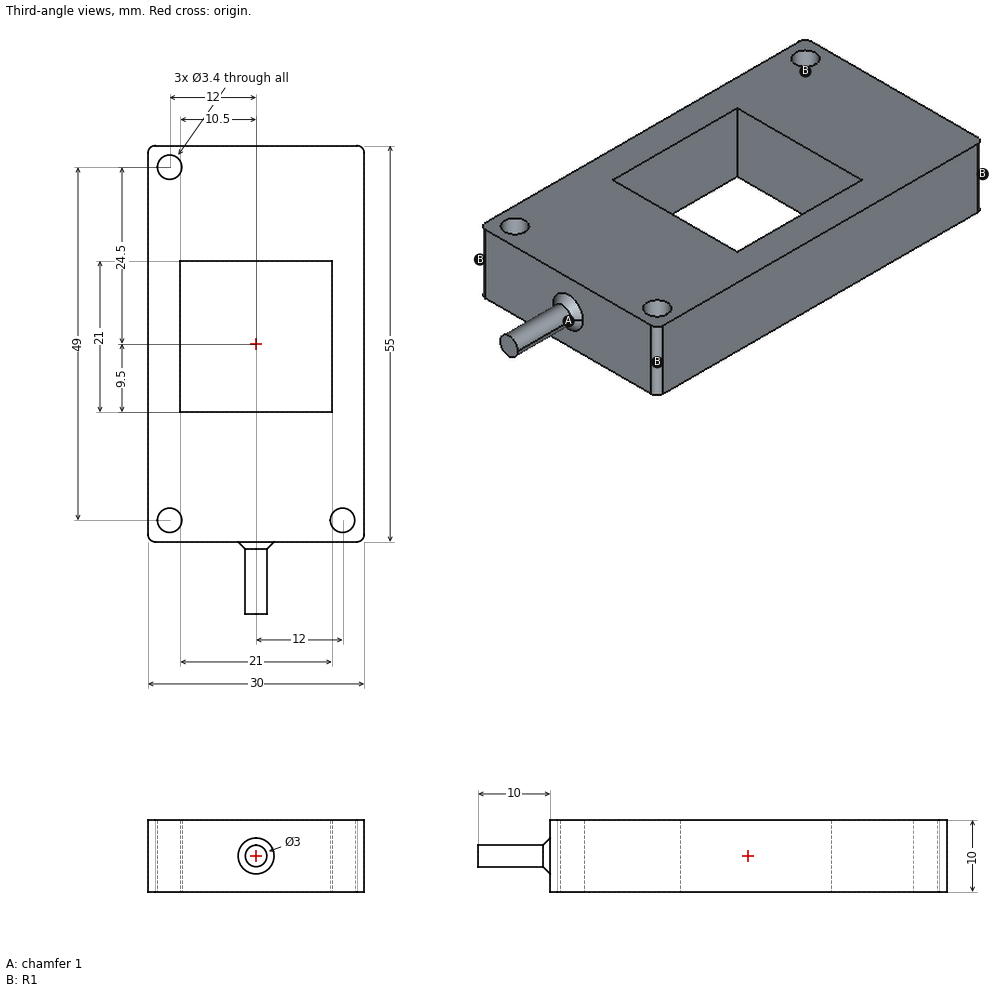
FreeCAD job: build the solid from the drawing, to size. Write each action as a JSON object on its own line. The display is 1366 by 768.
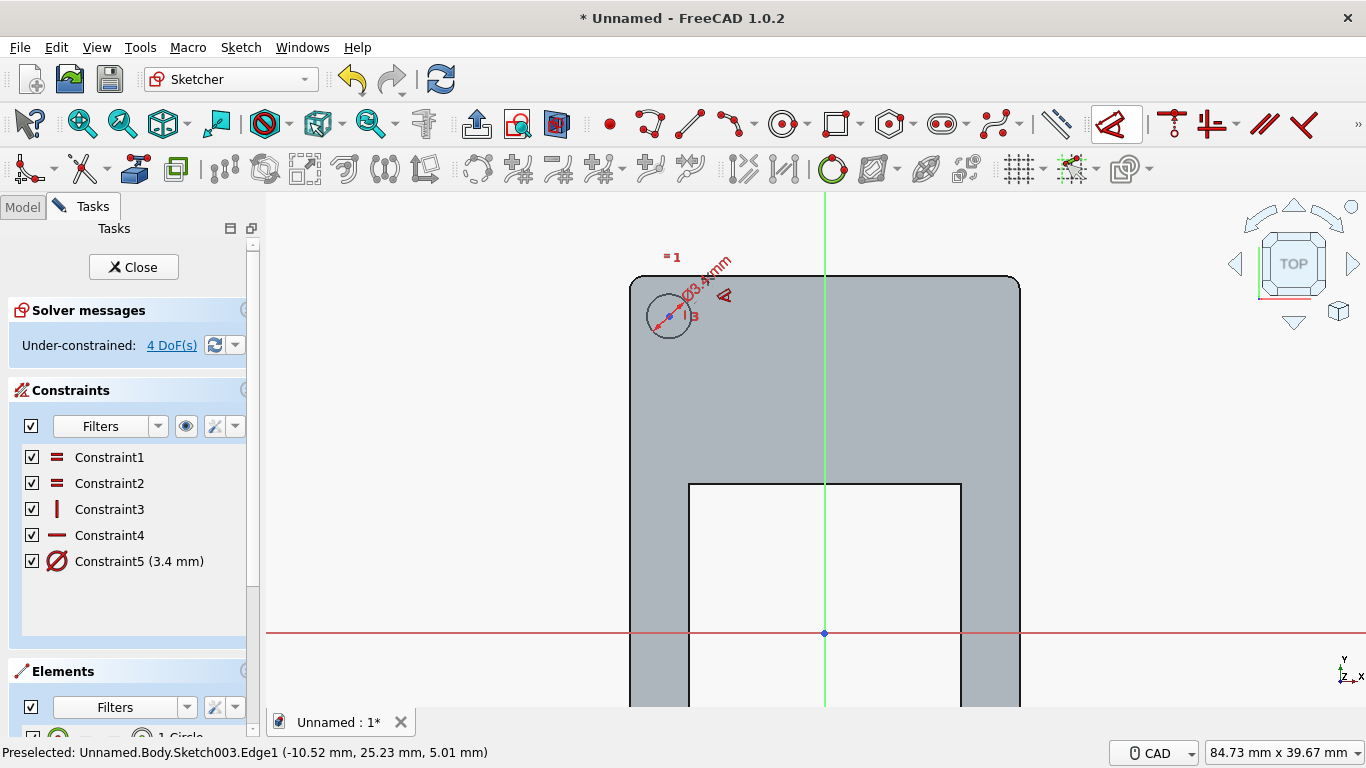
{"action": "left_click", "coordinate": [669, 316]}
{"action": "left_click", "coordinate": [783, 282]}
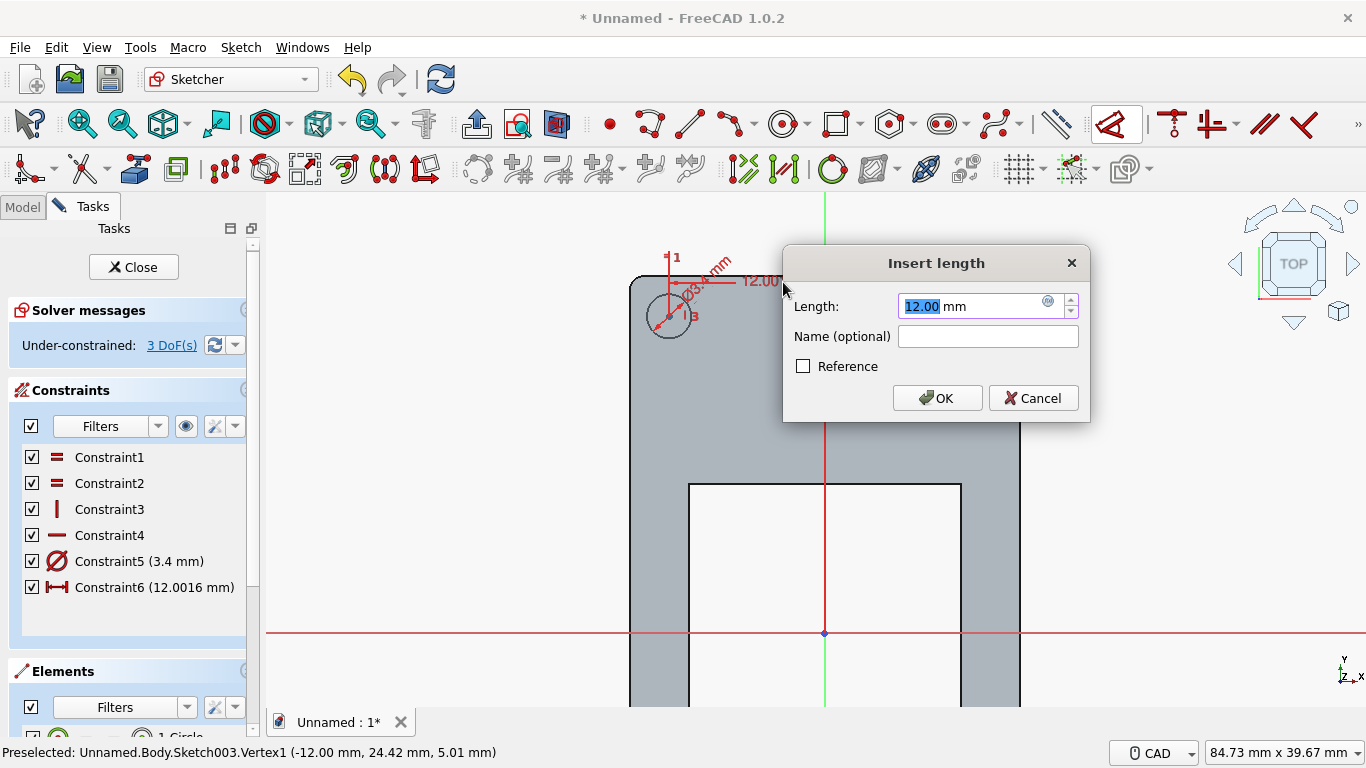
{"action": "type", "text": "12"}
{"action": "key", "text": "Return"}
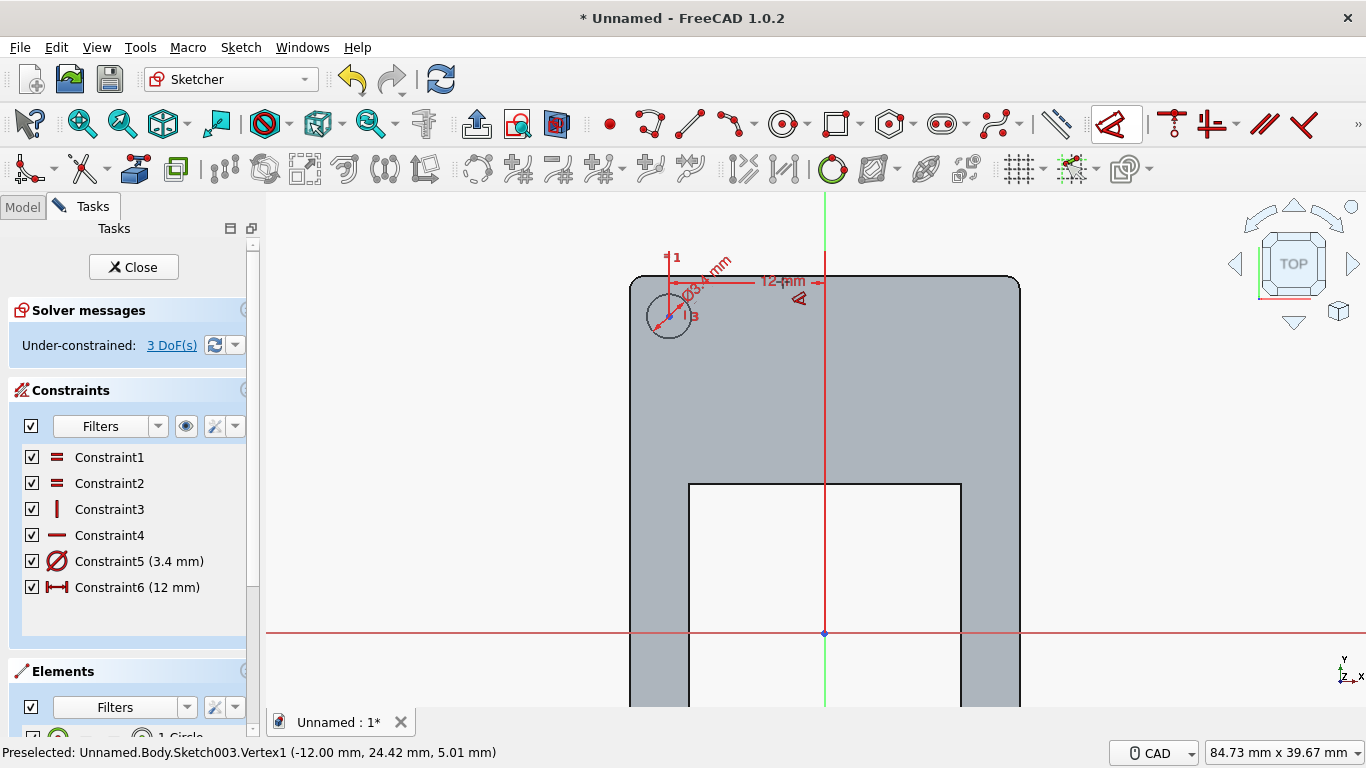
{"action": "scroll", "coordinate": [684, 300], "scroll_direction": "down", "scroll_amount": 4}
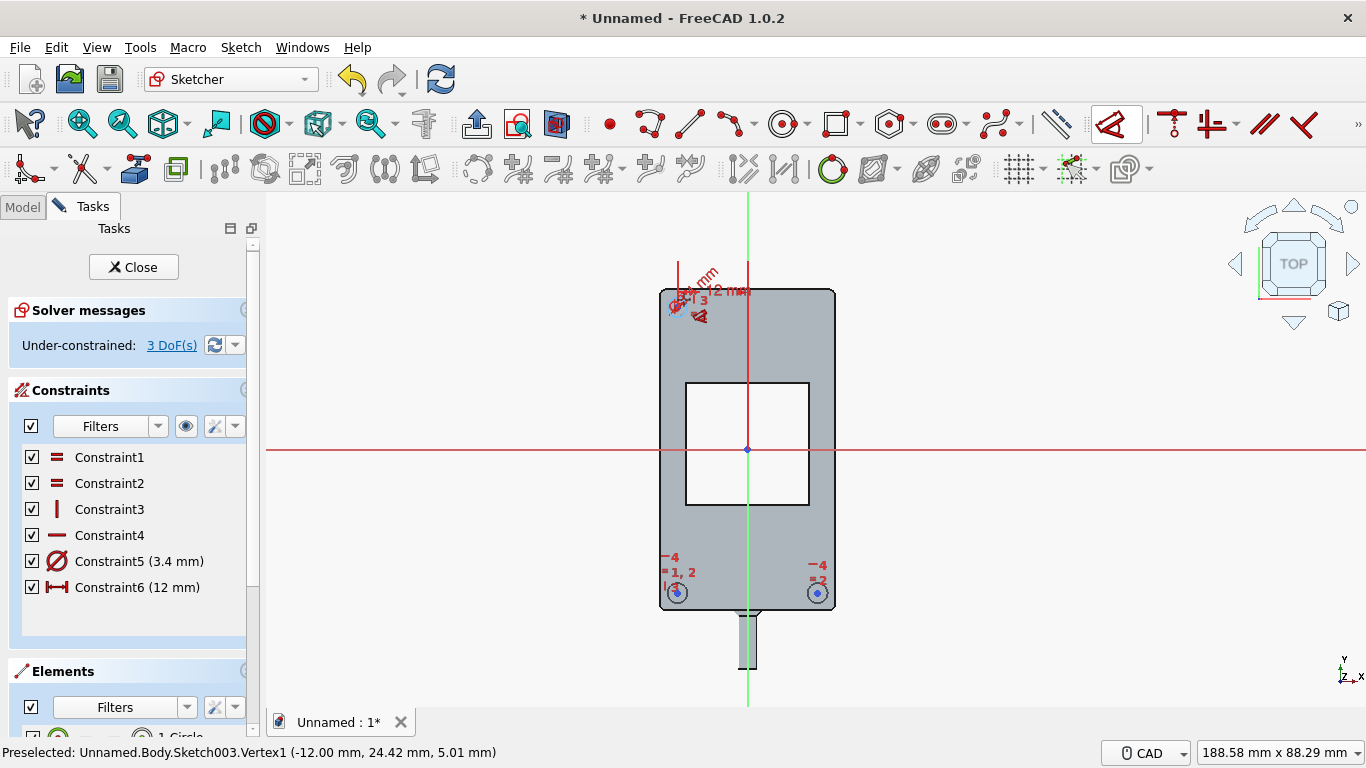
{"action": "left_click", "coordinate": [818, 593]}
{"action": "left_click", "coordinate": [783, 627]}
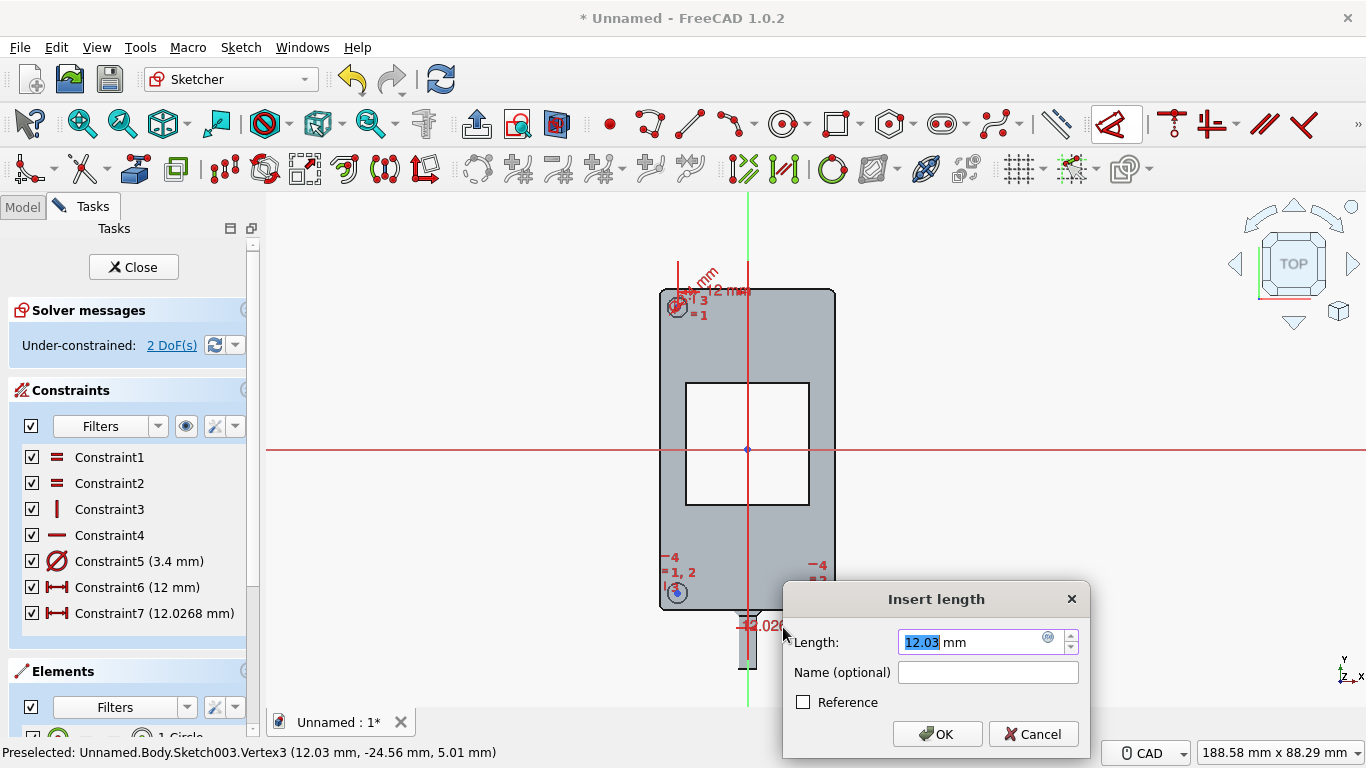
{"action": "type", "text": "12"}
{"action": "key", "text": "Return"}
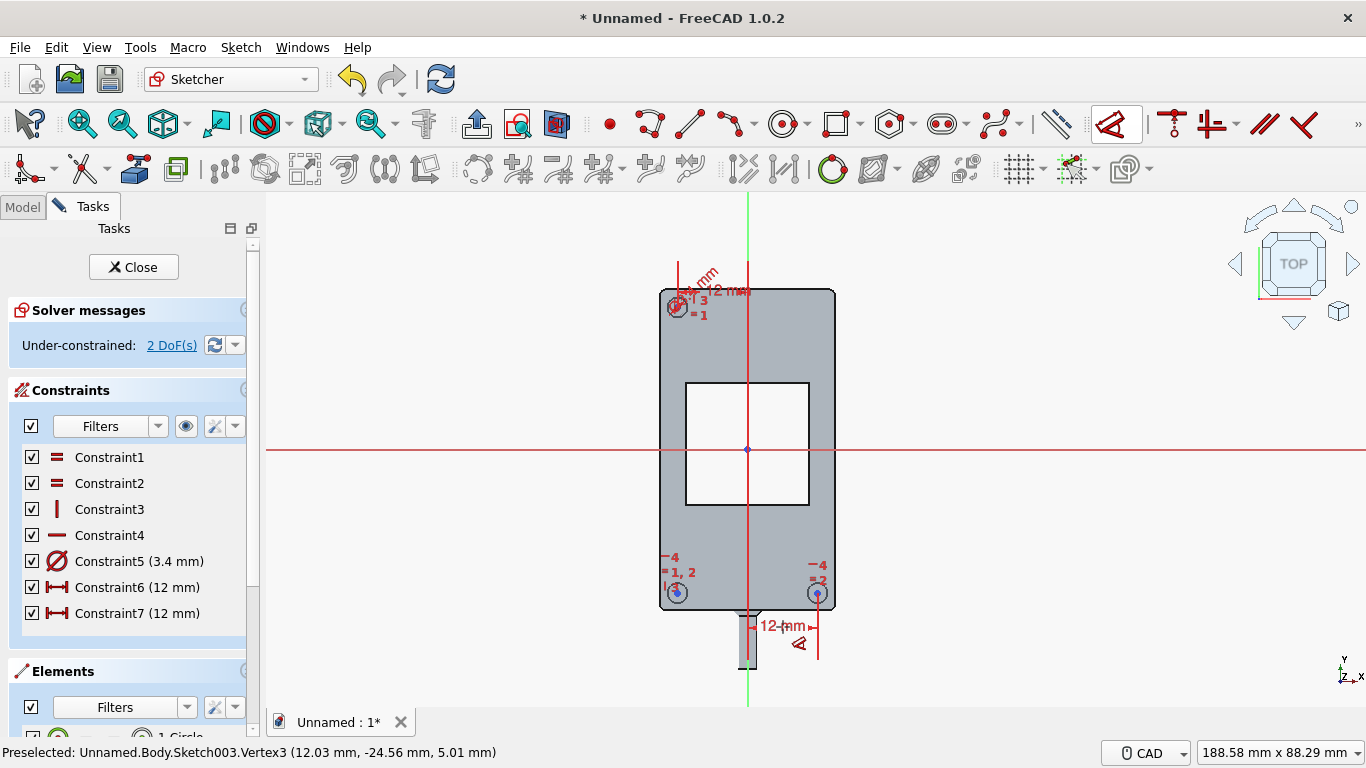
{"action": "left_click", "coordinate": [678, 307]}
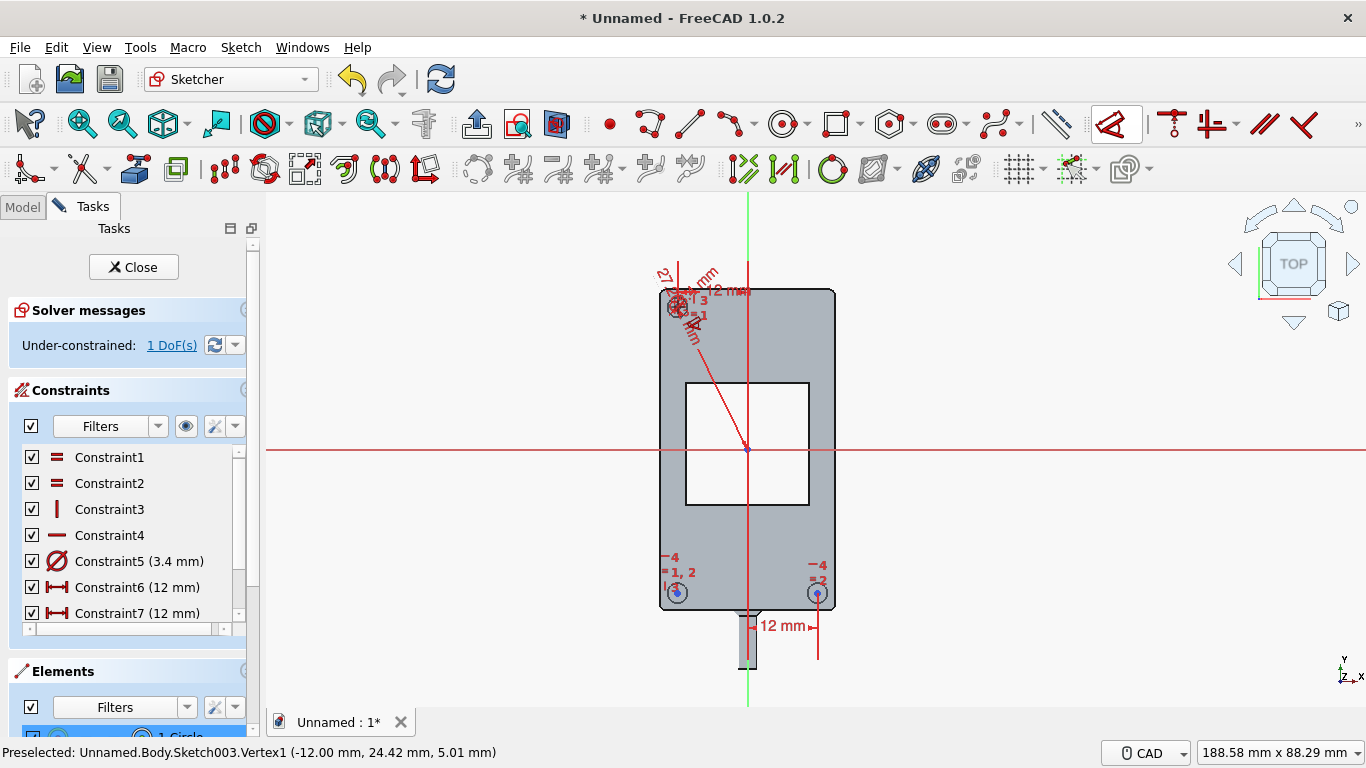
{"action": "left_click", "coordinate": [678, 593]}
{"action": "left_click", "coordinate": [644, 385]}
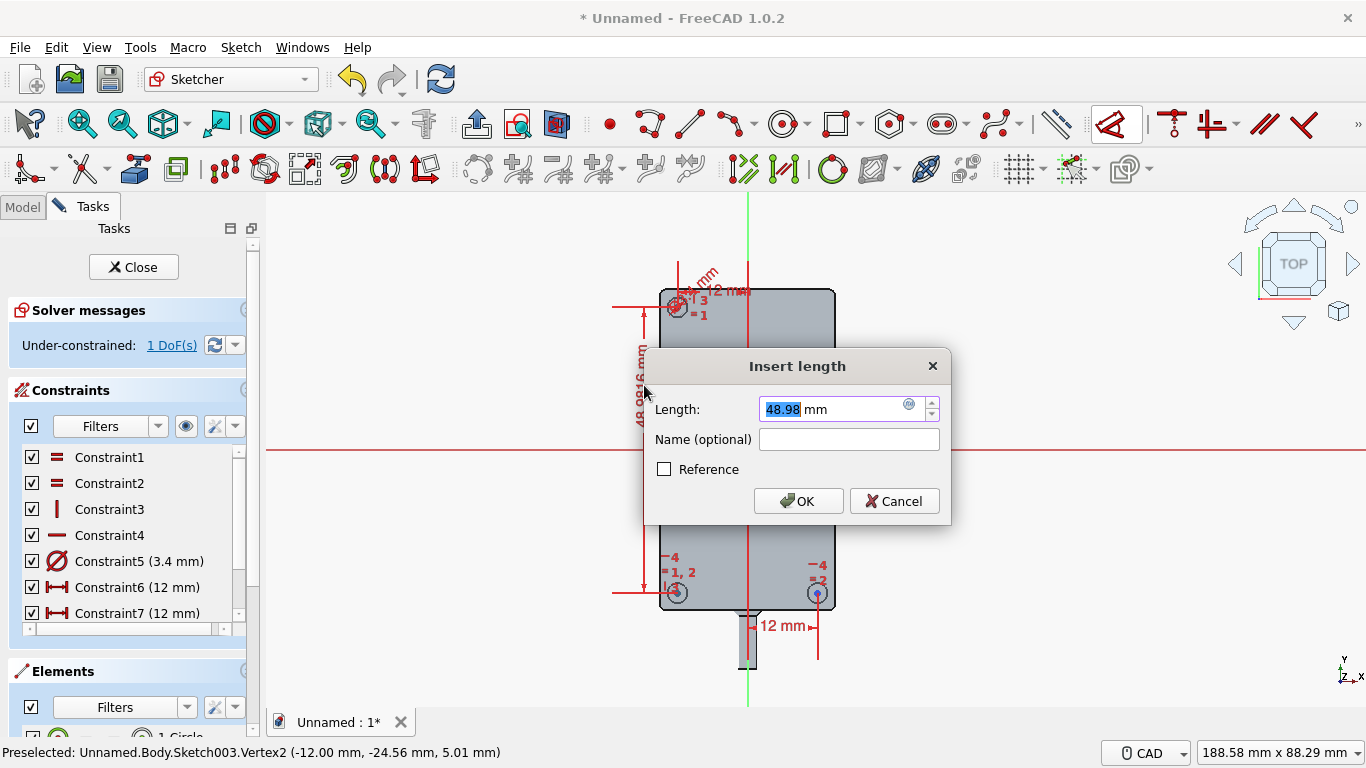
{"action": "type", "text": "49"}
{"action": "key", "text": "Return"}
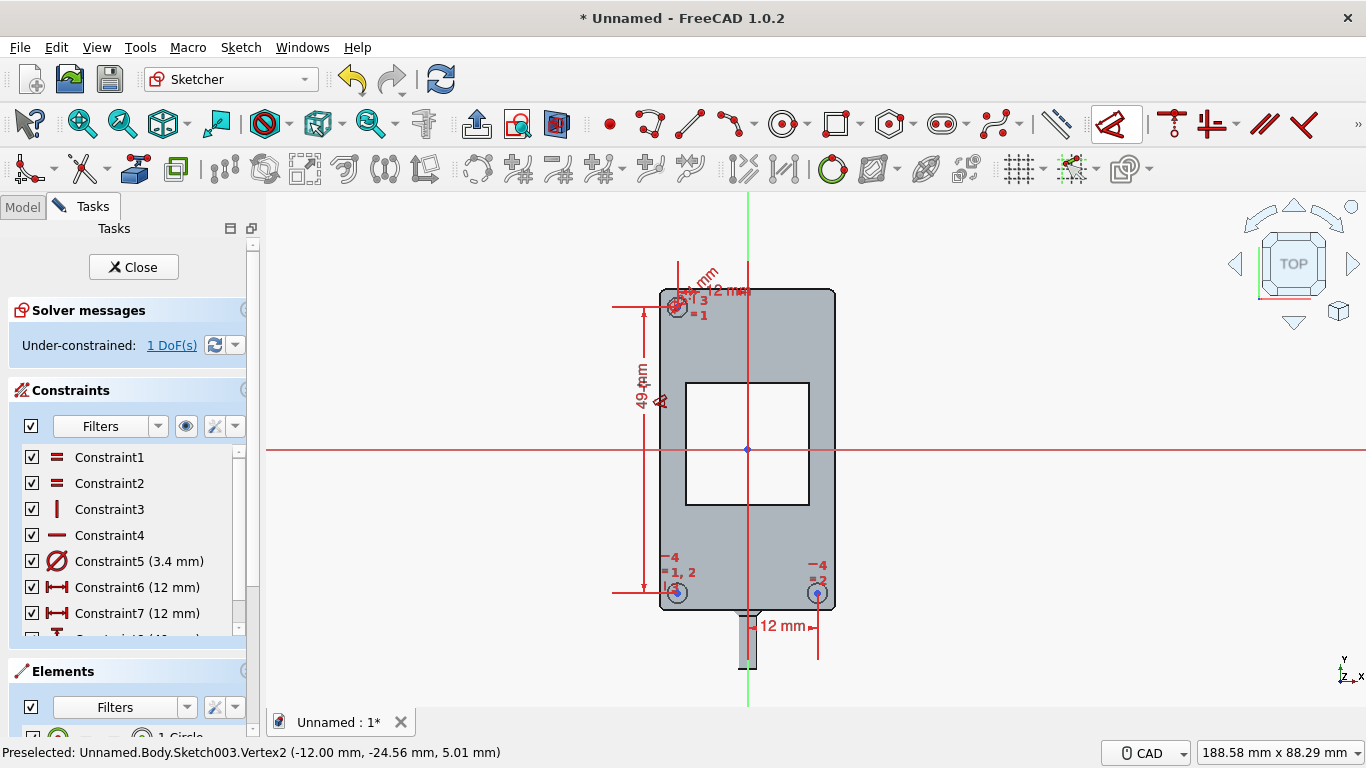
{"action": "left_click", "coordinate": [678, 307]}
{"action": "left_click", "coordinate": [644, 346]}